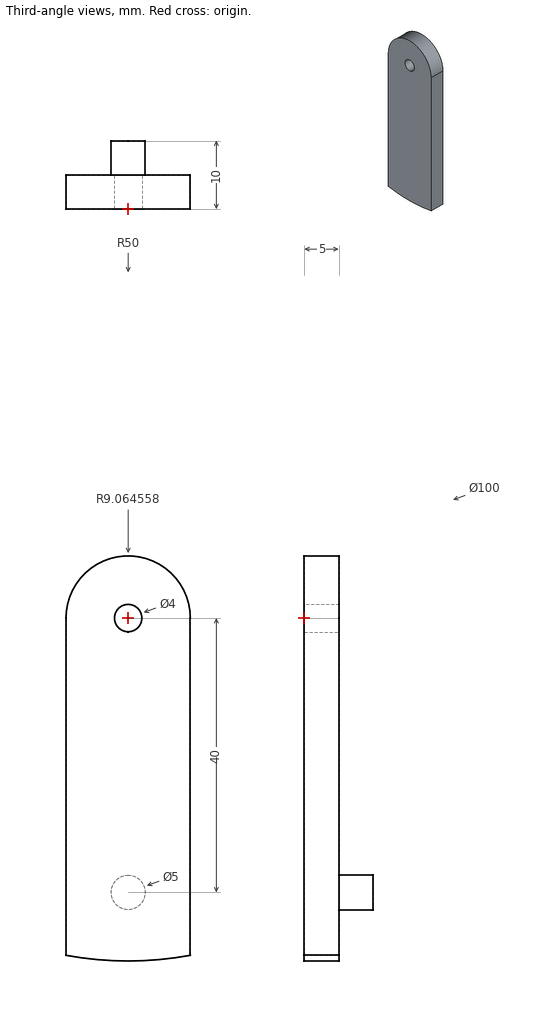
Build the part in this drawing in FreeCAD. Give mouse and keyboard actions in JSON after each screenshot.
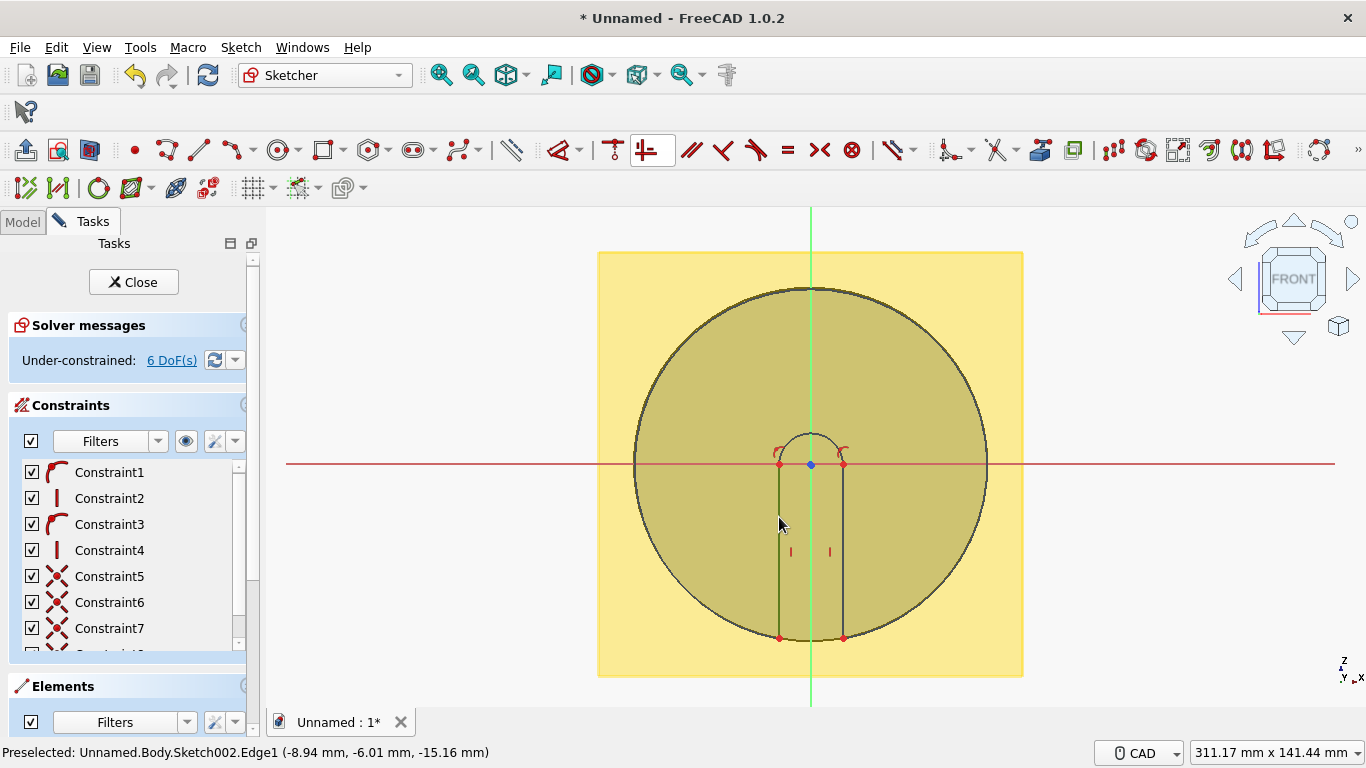
{"action": "left_click", "coordinate": [829, 439]}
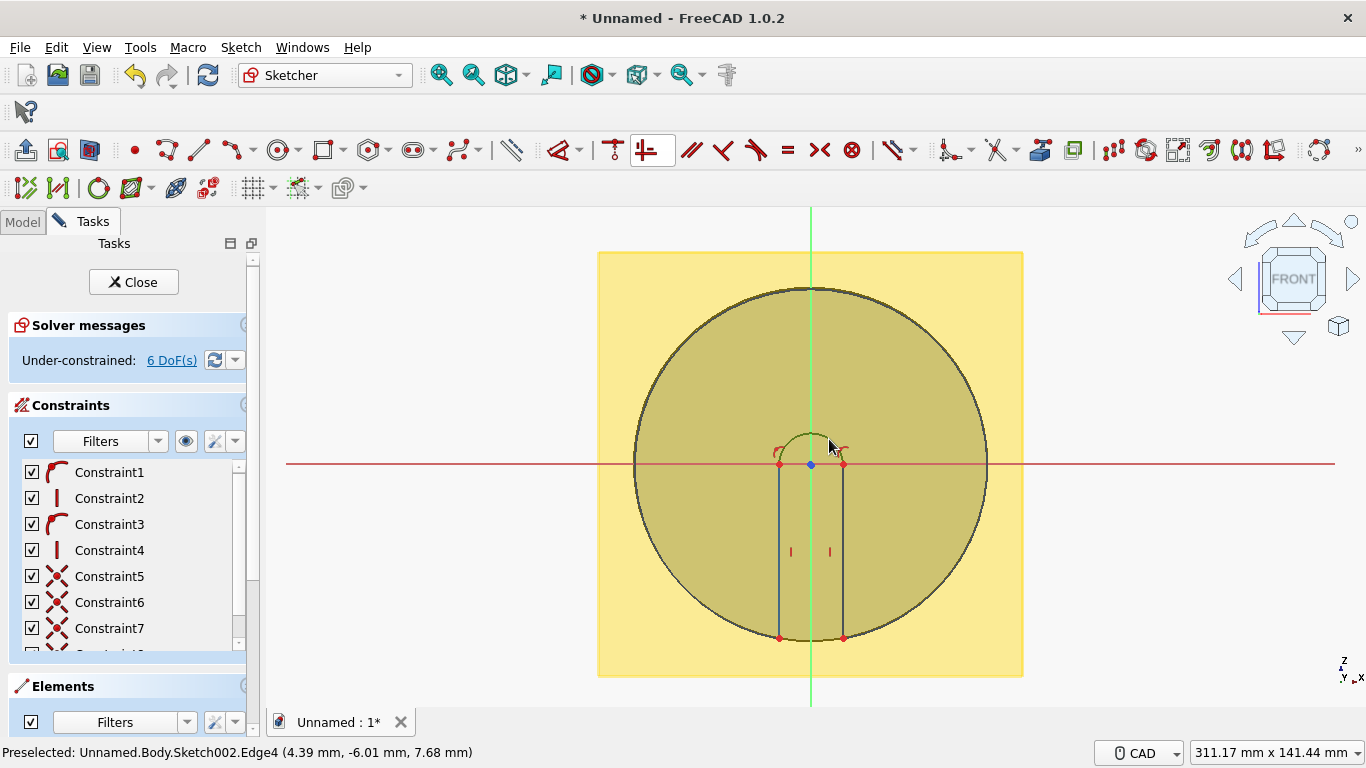
{"action": "left_click", "coordinate": [756, 150]}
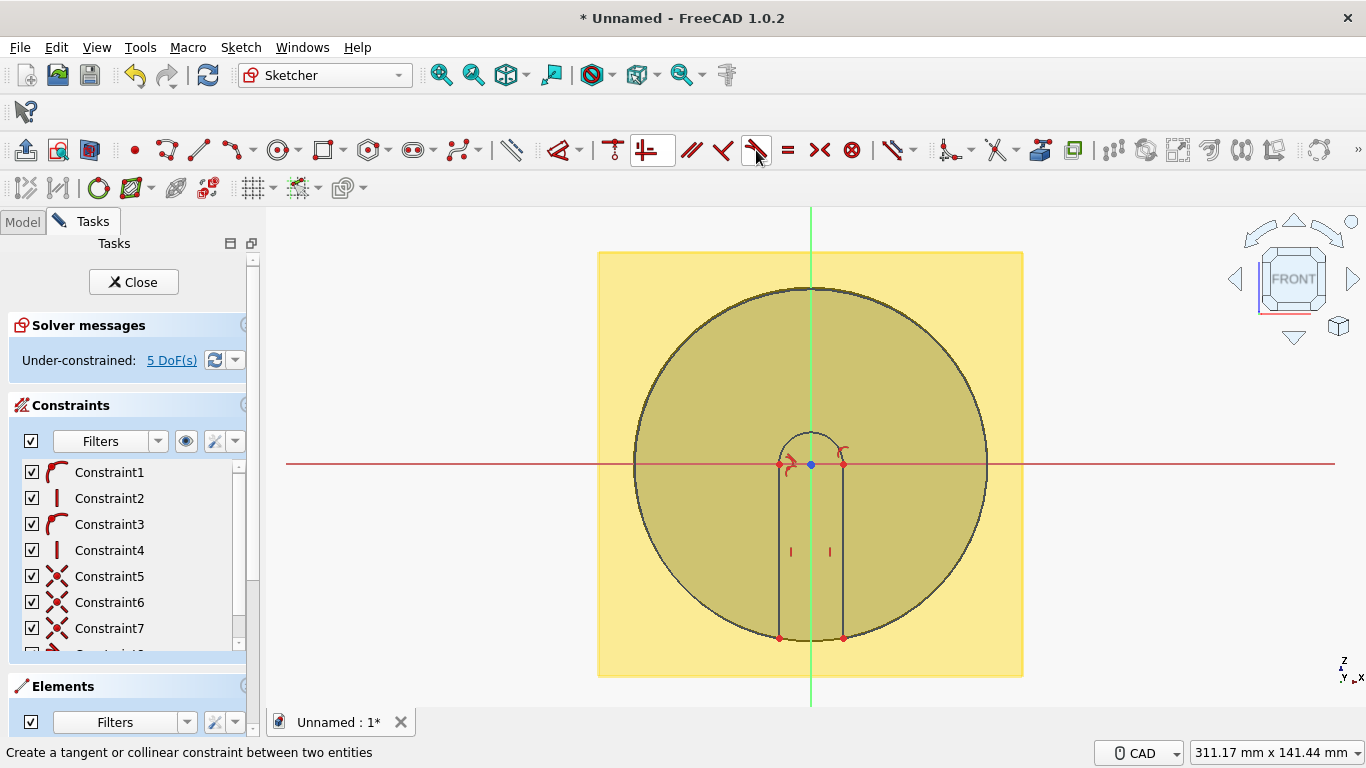
{"action": "left_click", "coordinate": [974, 399]}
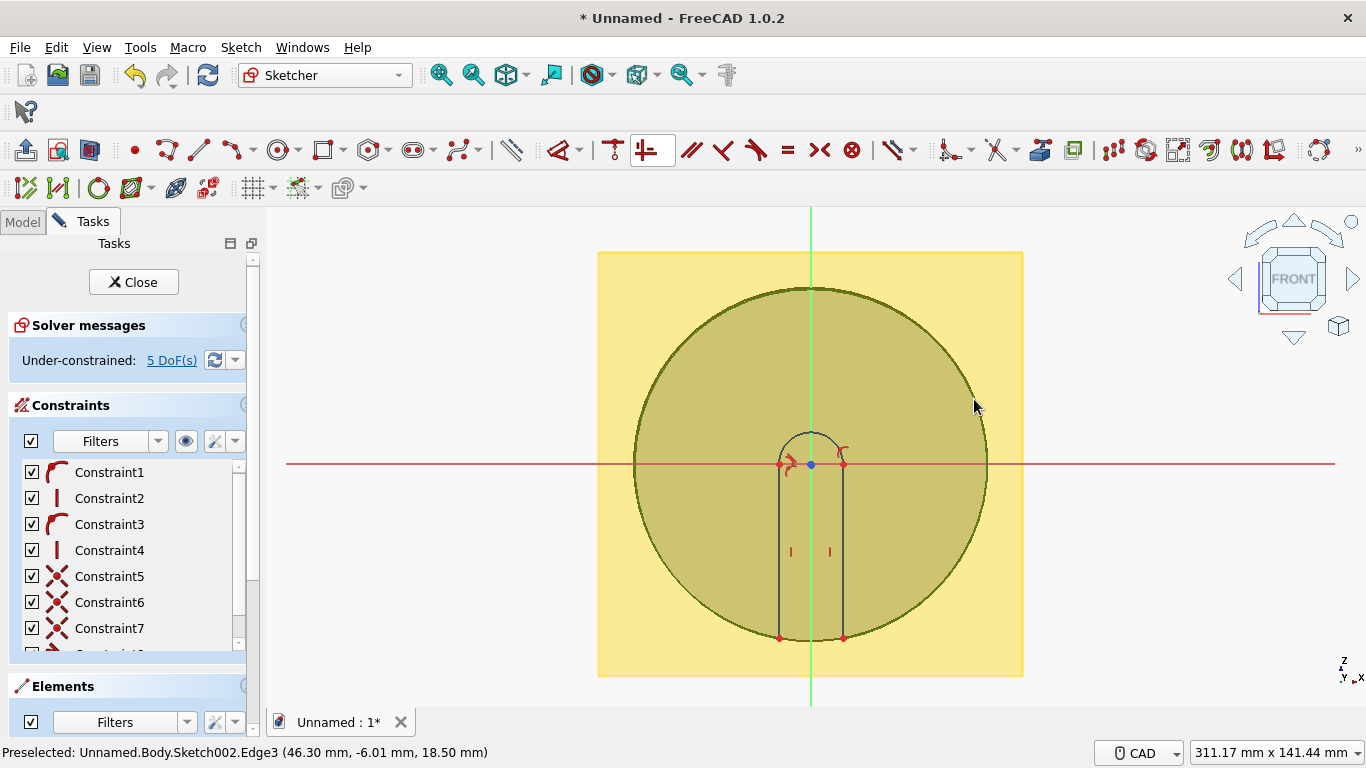
{"action": "left_click", "coordinate": [830, 439]}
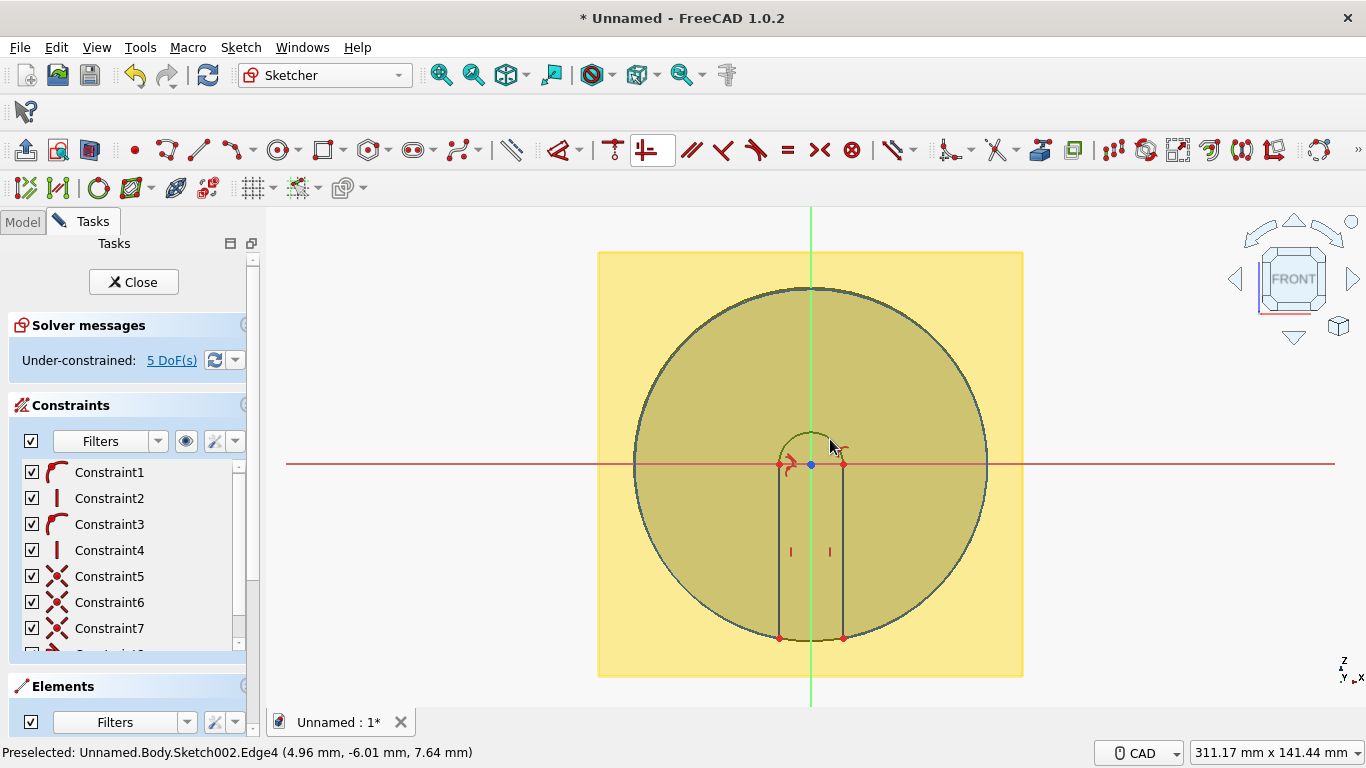
{"action": "left_click", "coordinate": [614, 150]}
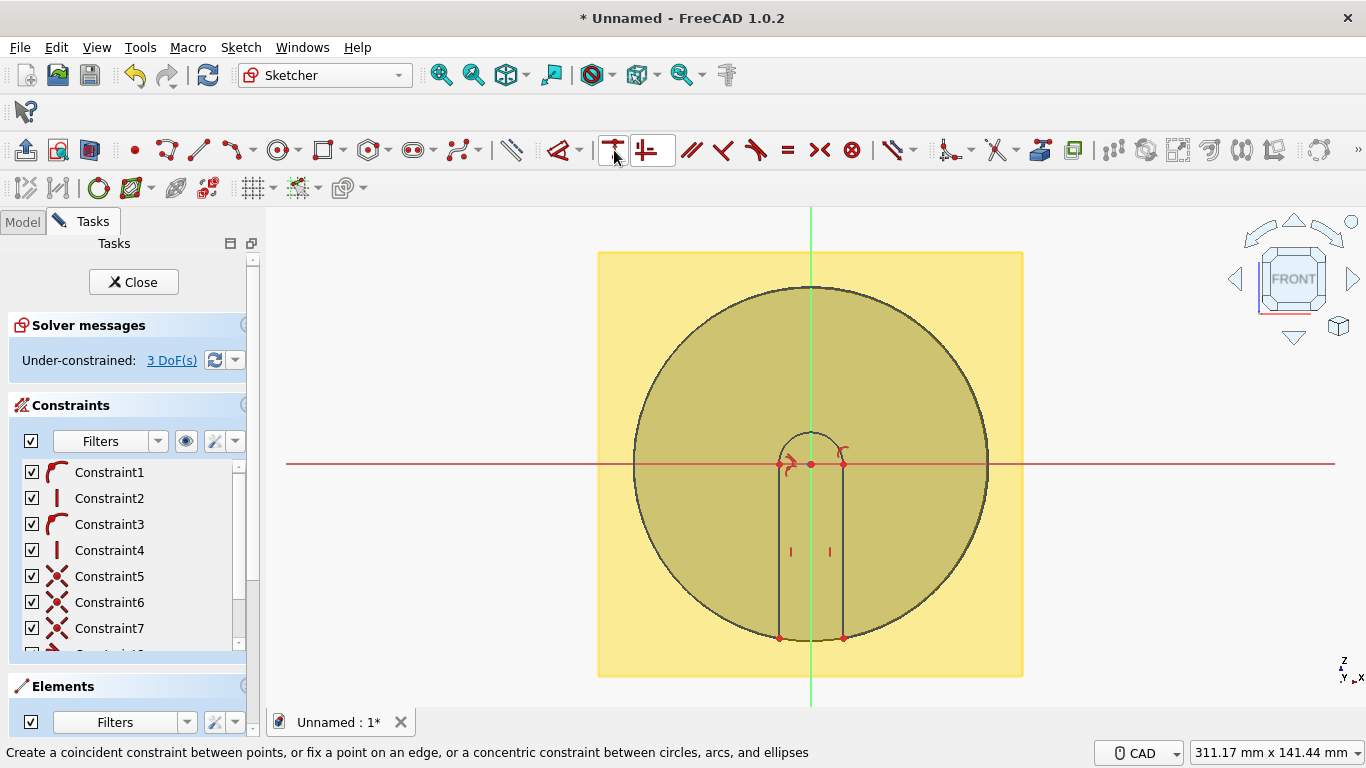
{"action": "left_click", "coordinate": [811, 464]}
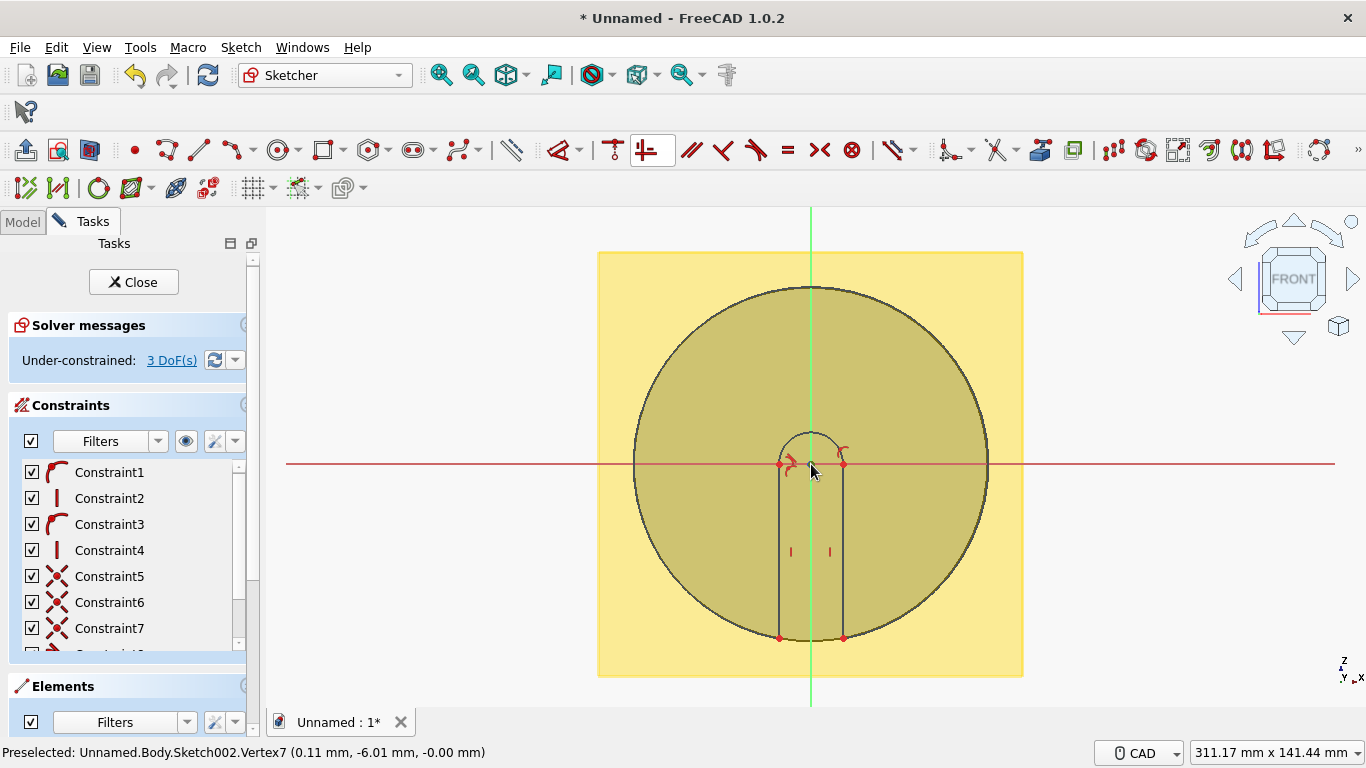
{"action": "left_click", "coordinate": [811, 647]}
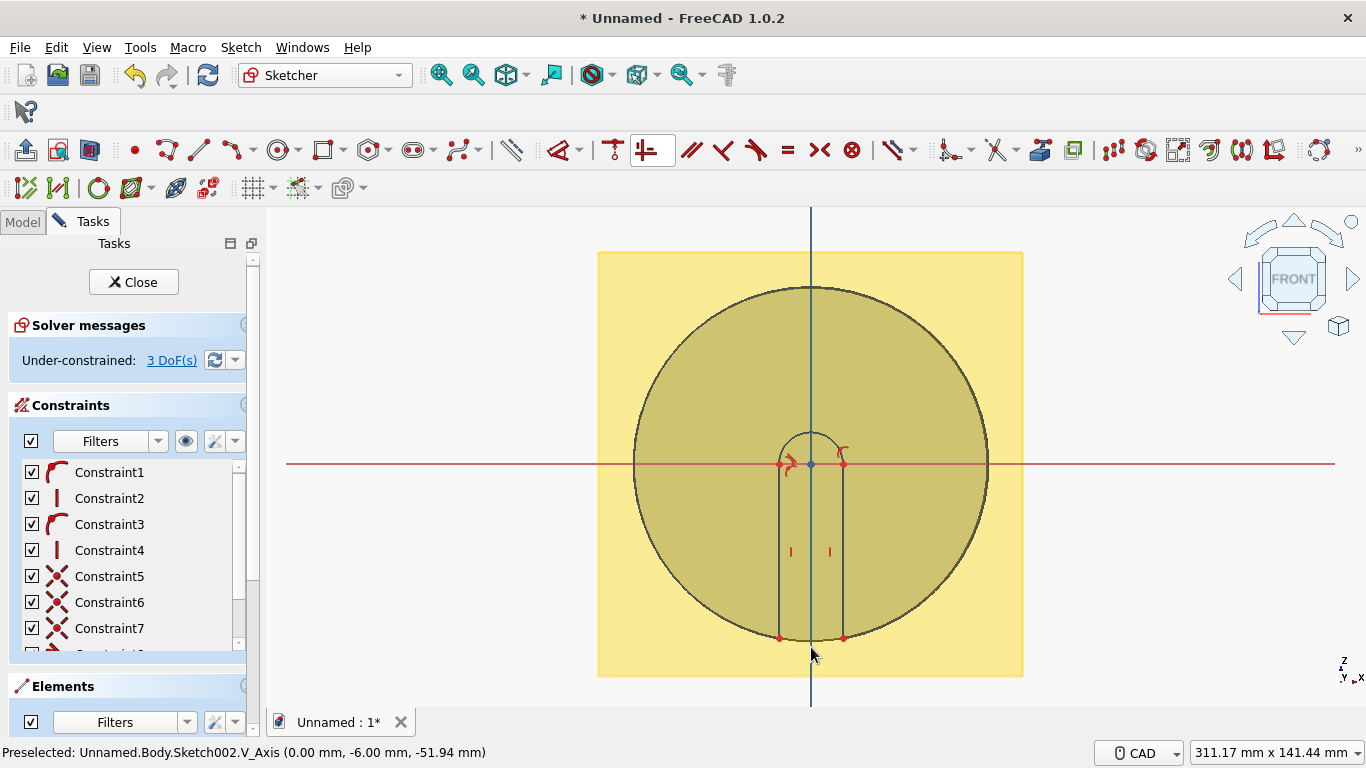
{"action": "left_click", "coordinate": [614, 150]}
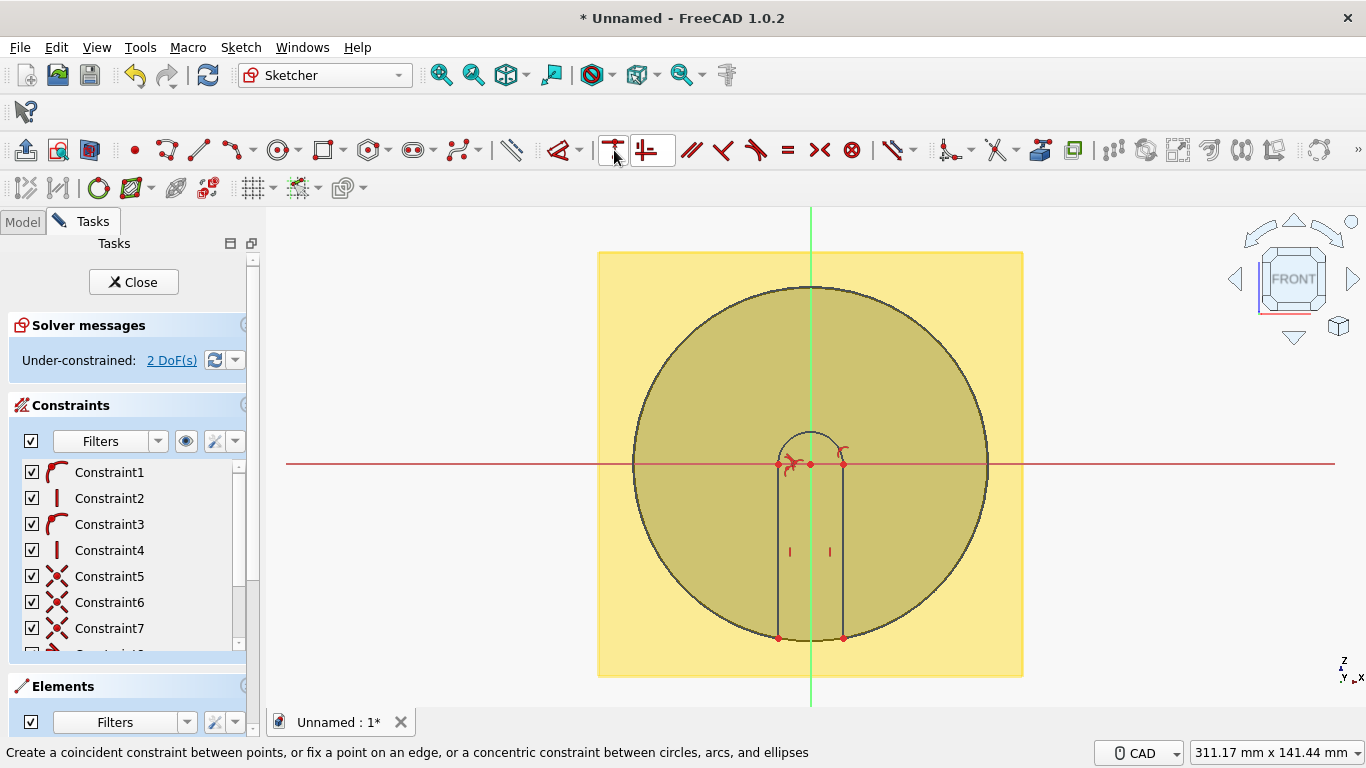
{"action": "left_click", "coordinate": [975, 397]}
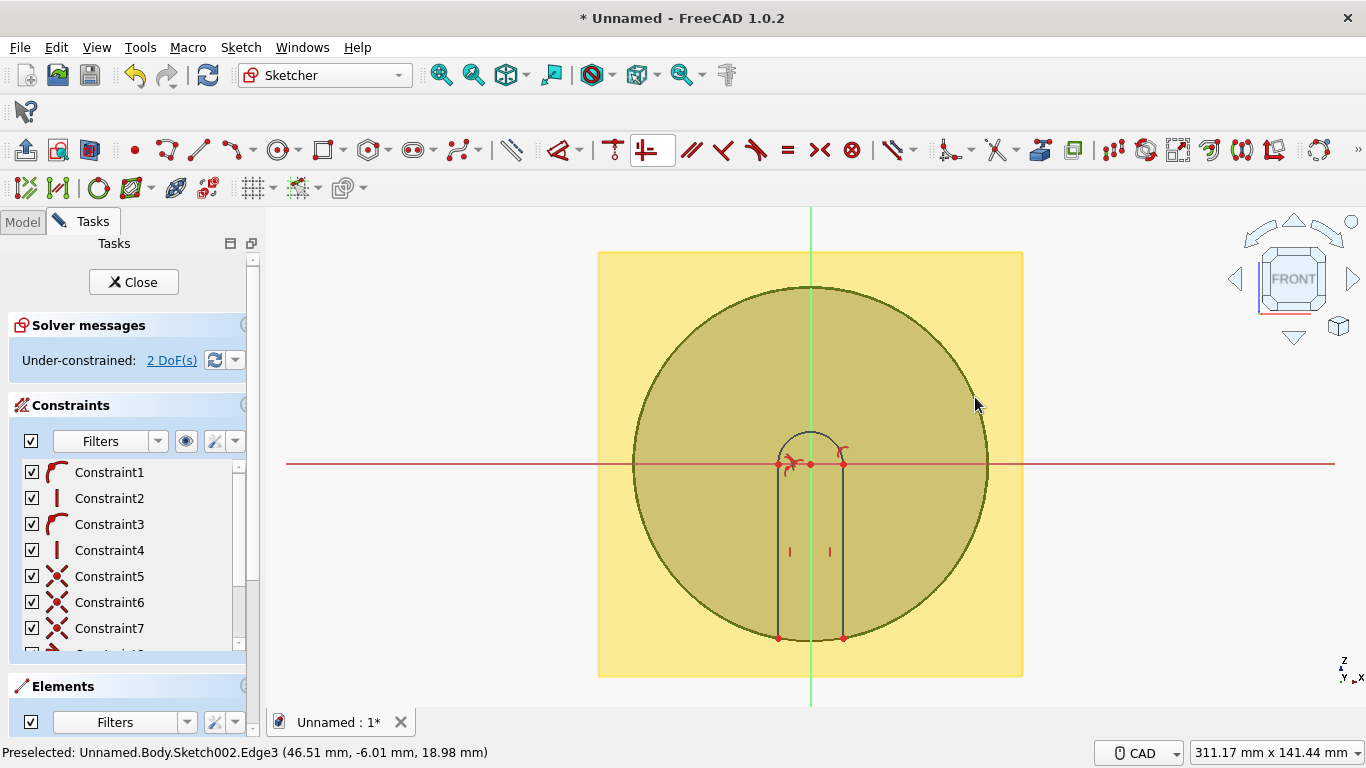
{"action": "key", "text": "k r"}